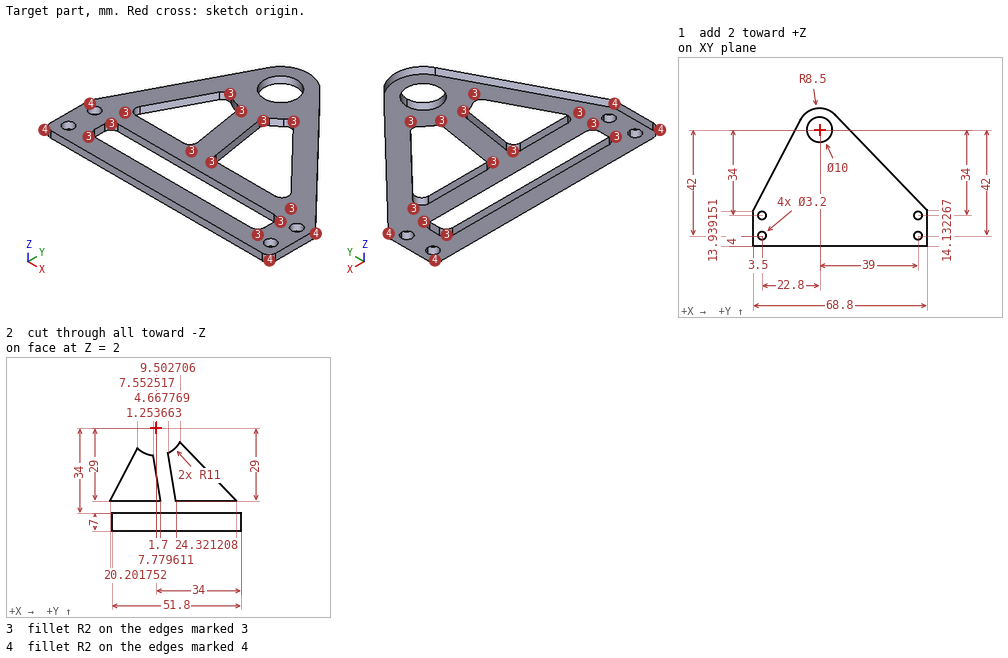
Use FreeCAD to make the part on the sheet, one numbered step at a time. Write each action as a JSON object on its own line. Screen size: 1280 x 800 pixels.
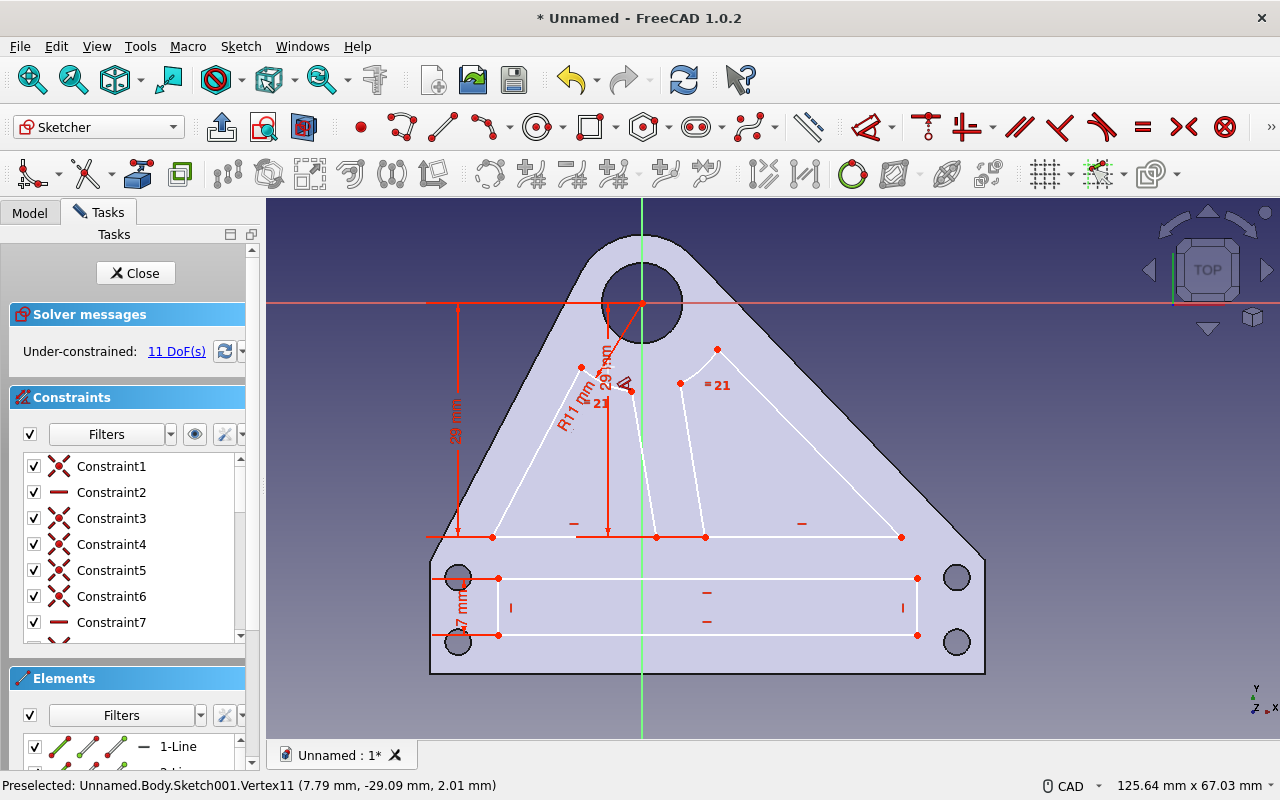
{"action": "left_click", "coordinate": [498, 579]}
{"action": "left_click", "coordinate": [464, 441]}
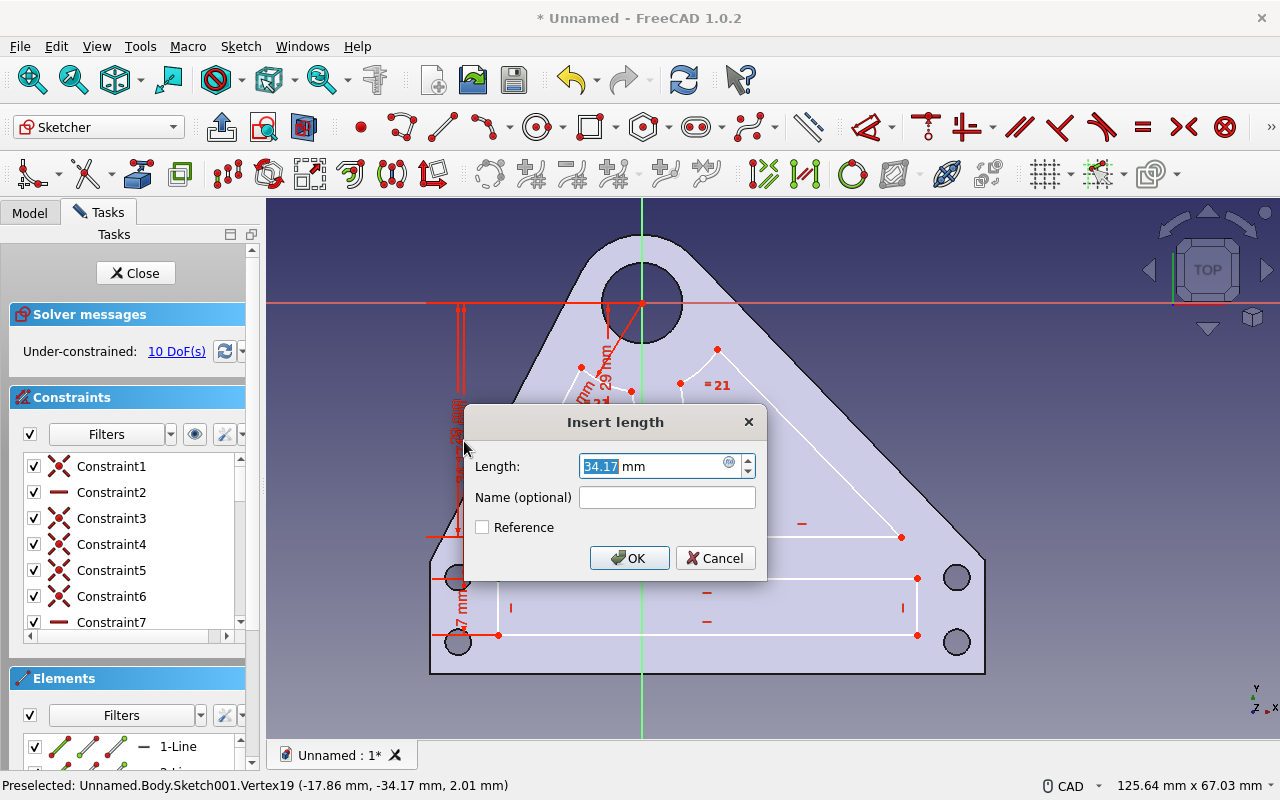
{"action": "type", "text": "34"}
{"action": "key", "text": "Return"}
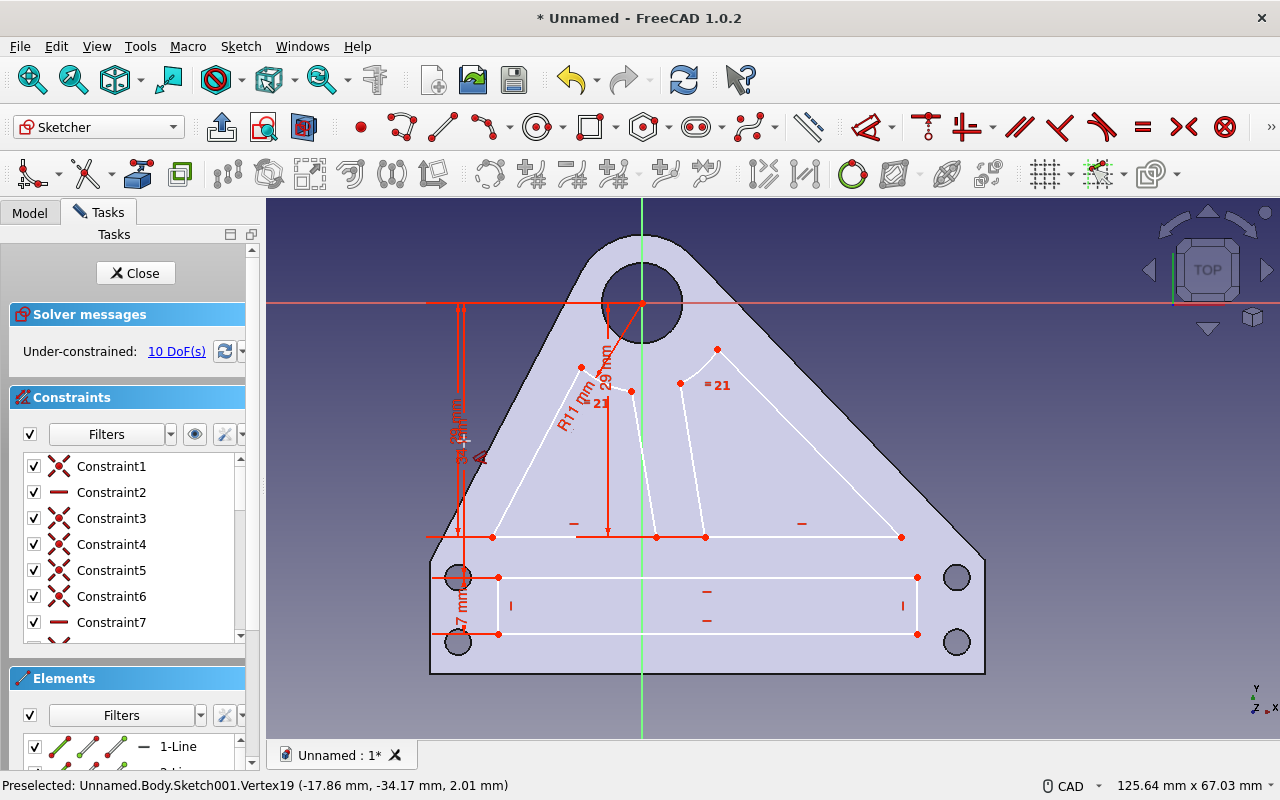
{"action": "left_click", "coordinate": [917, 634]}
{"action": "left_click", "coordinate": [780, 668]}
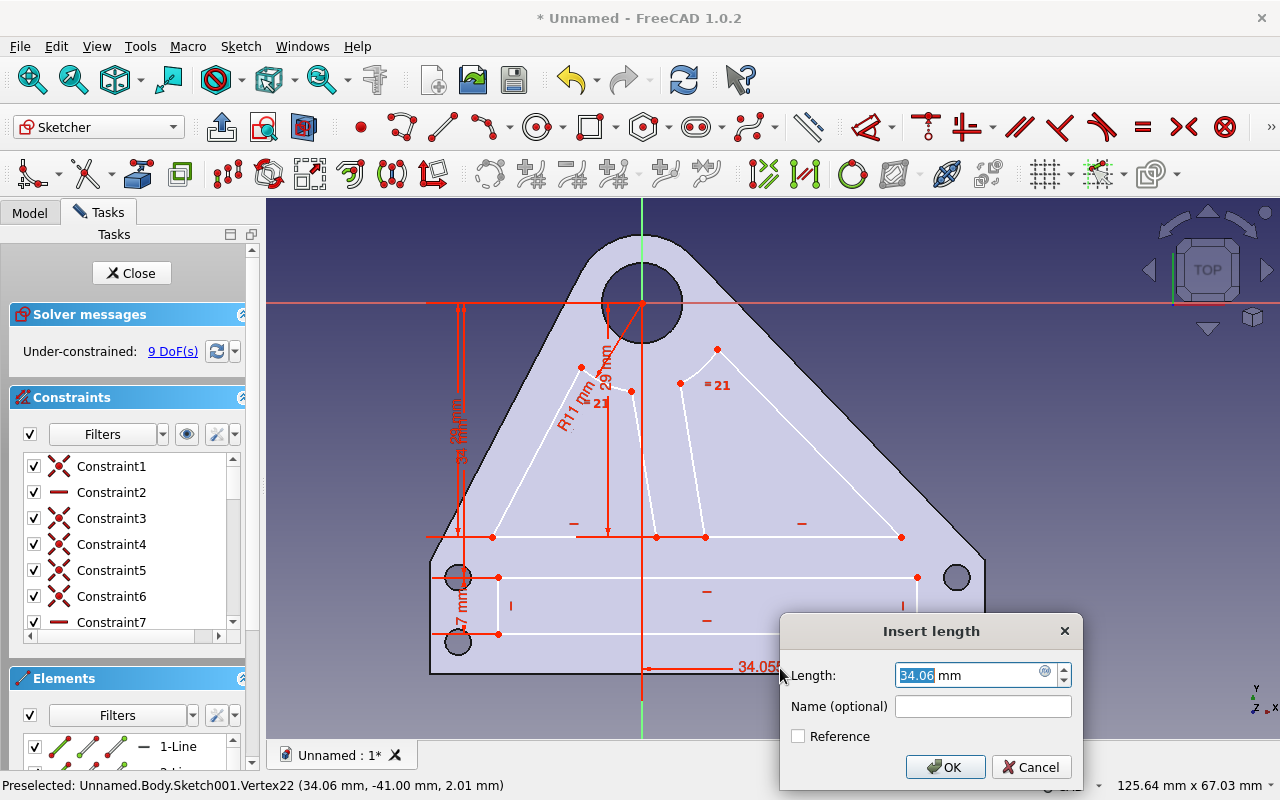
{"action": "type", "text": "34"}
{"action": "key", "text": "Return"}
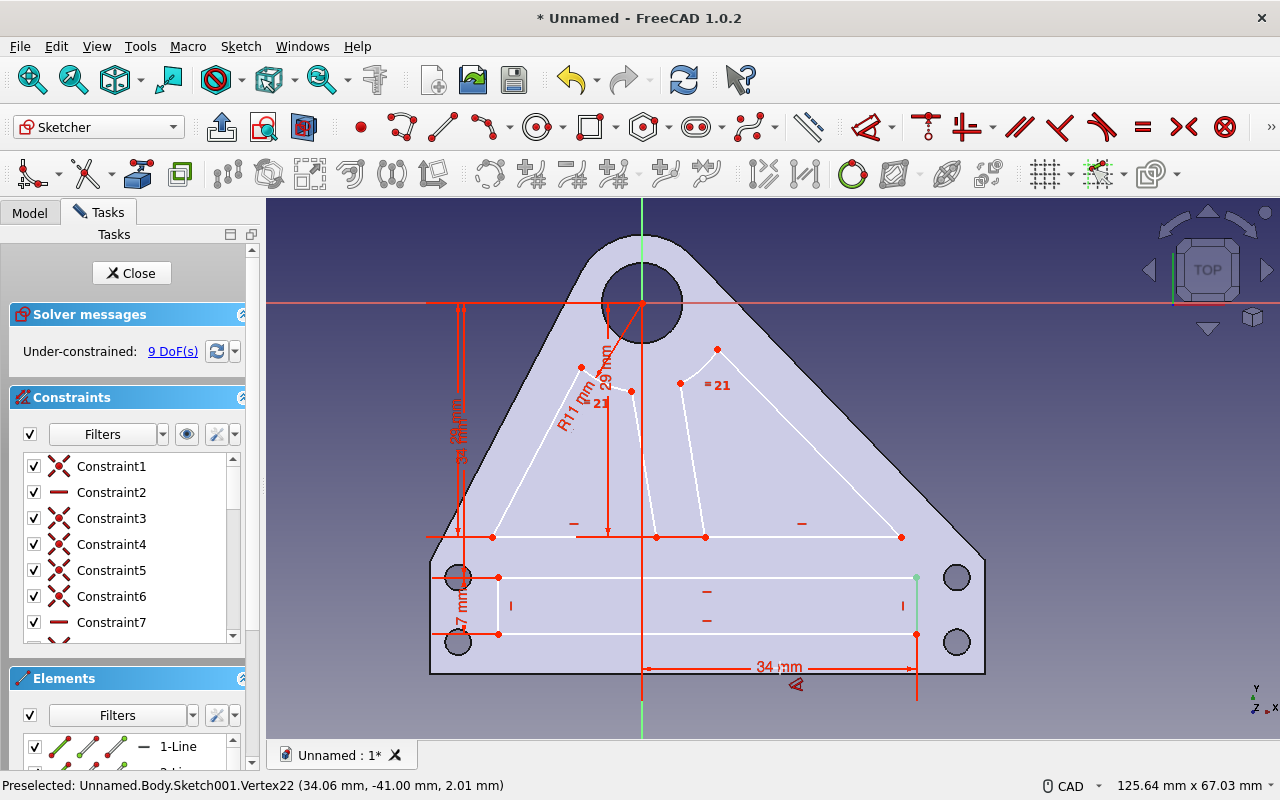
{"action": "left_click", "coordinate": [624, 634]}
{"action": "left_click", "coordinate": [707, 668]}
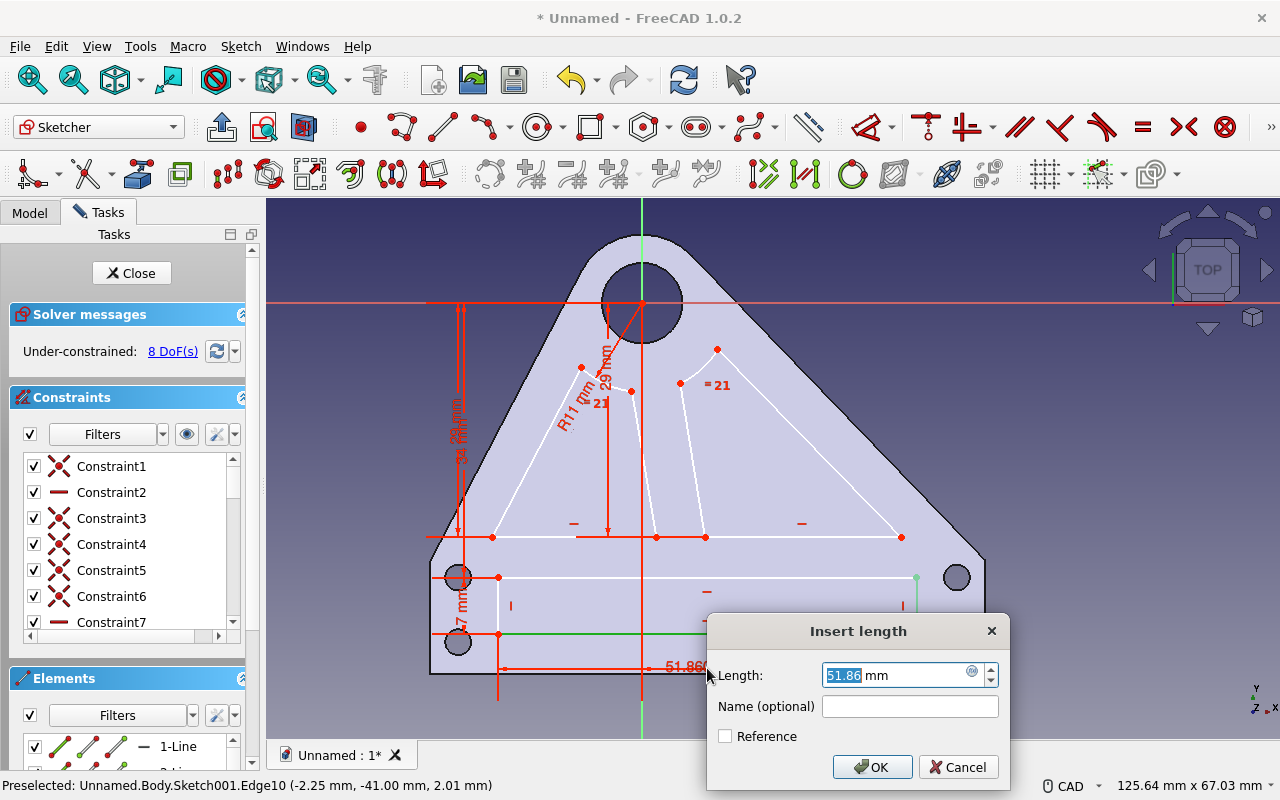
{"action": "type", "text": "51.8"}
{"action": "key", "text": "Return"}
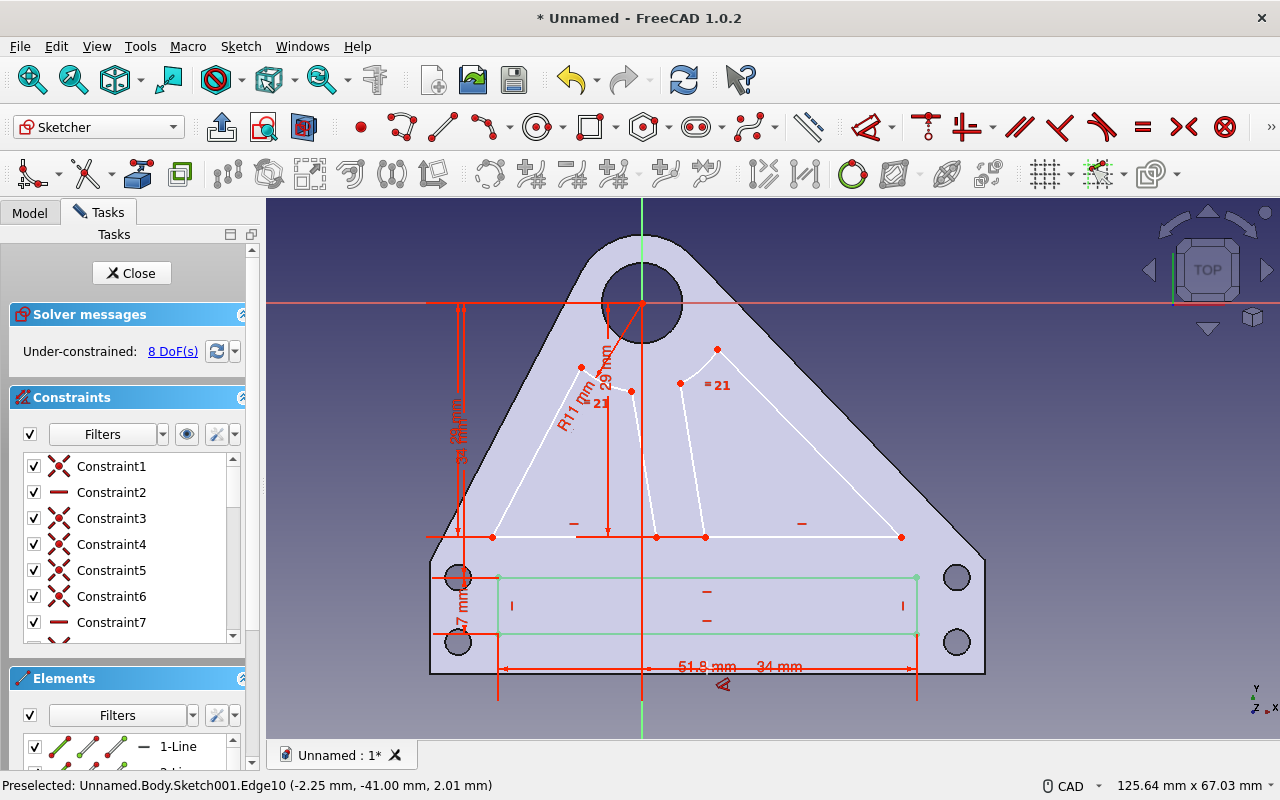
{"action": "scroll", "coordinate": [656, 537], "scroll_direction": "up", "scroll_amount": 6}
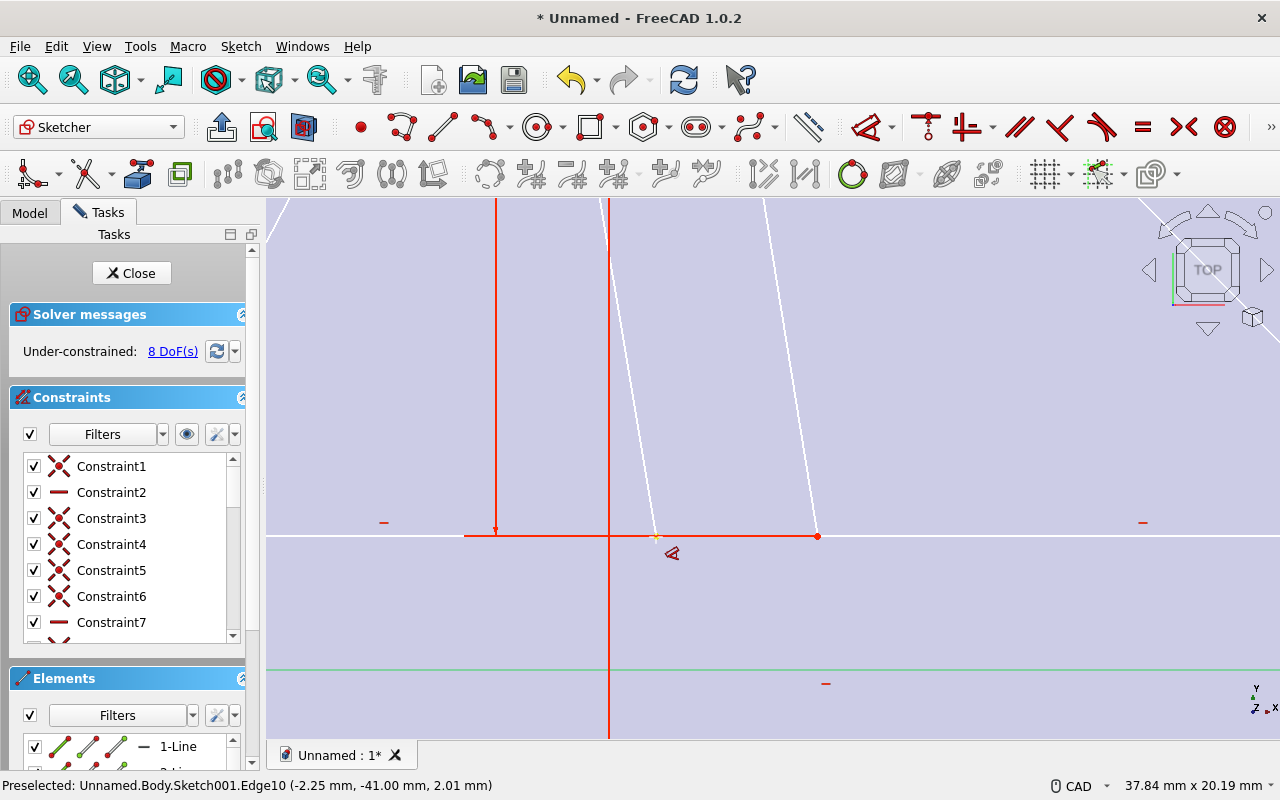
{"action": "left_click", "coordinate": [656, 536]}
{"action": "left_click", "coordinate": [633, 570]}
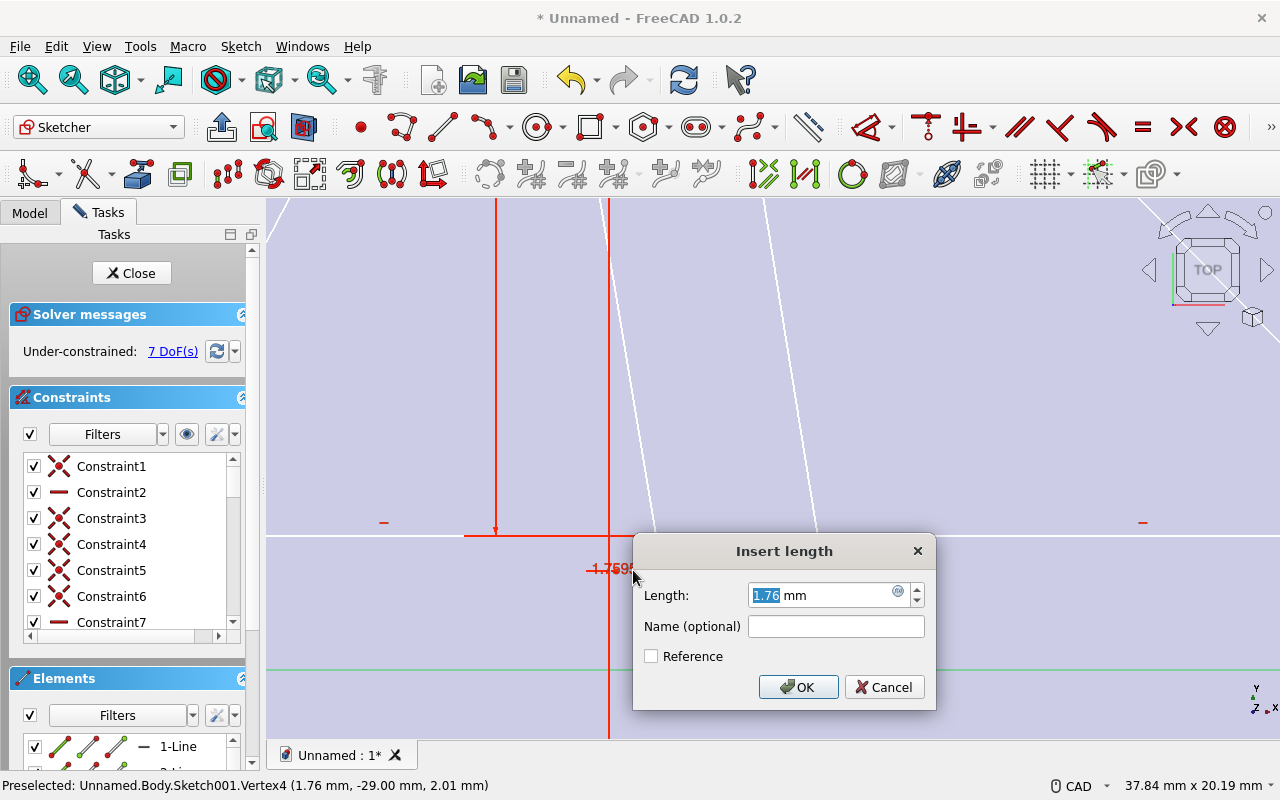
{"action": "type", "text": "1.7"}
{"action": "key", "text": "Return"}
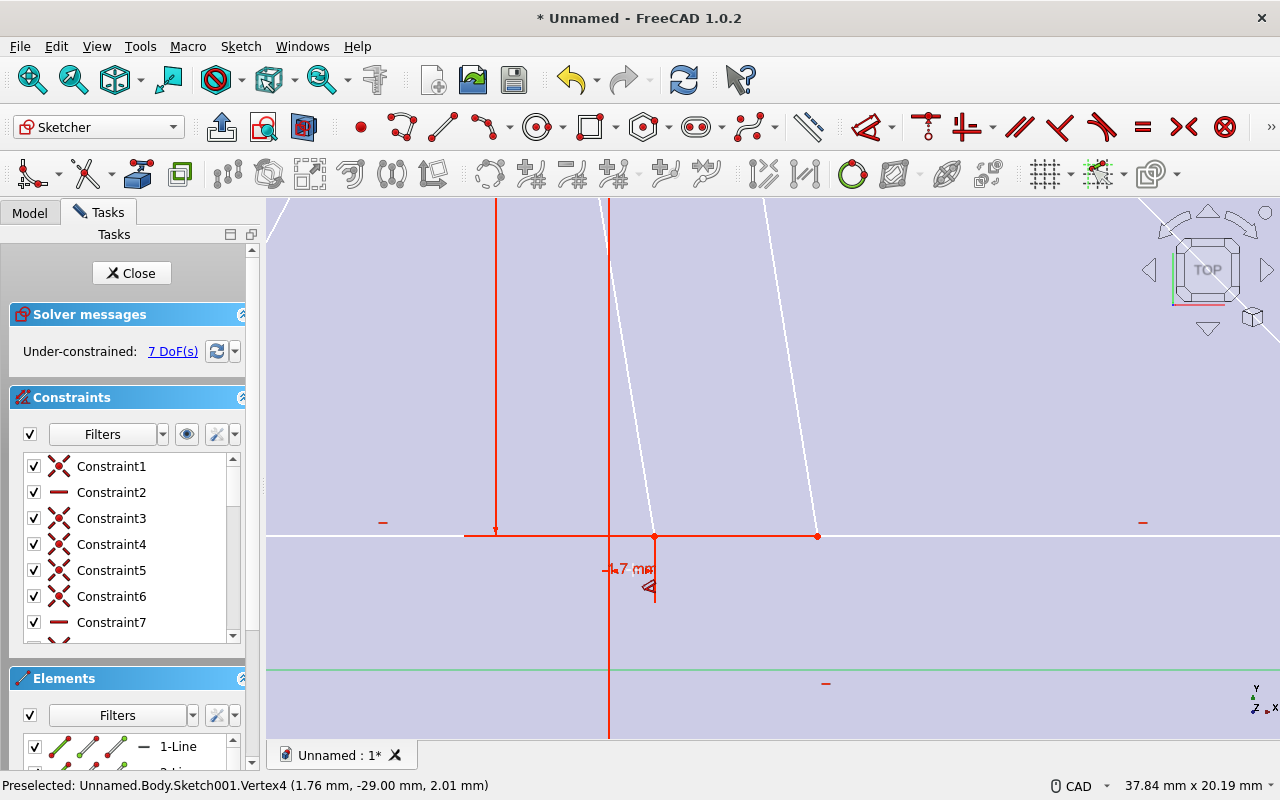
{"action": "left_click", "coordinate": [492, 536]}
{"action": "left_click", "coordinate": [474, 570]}